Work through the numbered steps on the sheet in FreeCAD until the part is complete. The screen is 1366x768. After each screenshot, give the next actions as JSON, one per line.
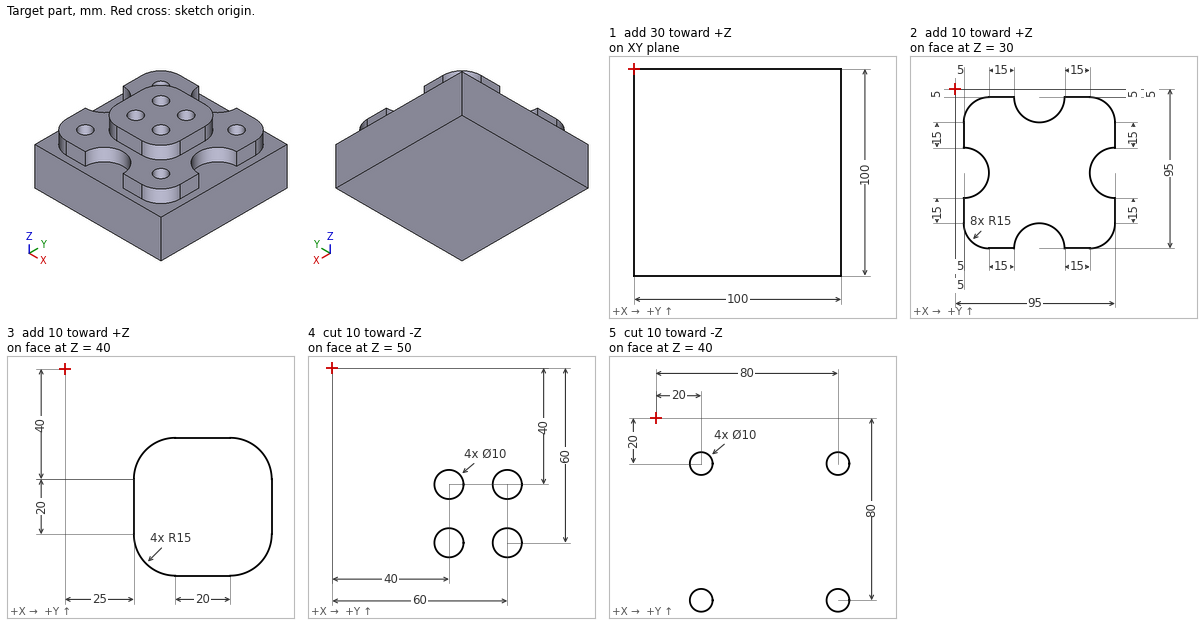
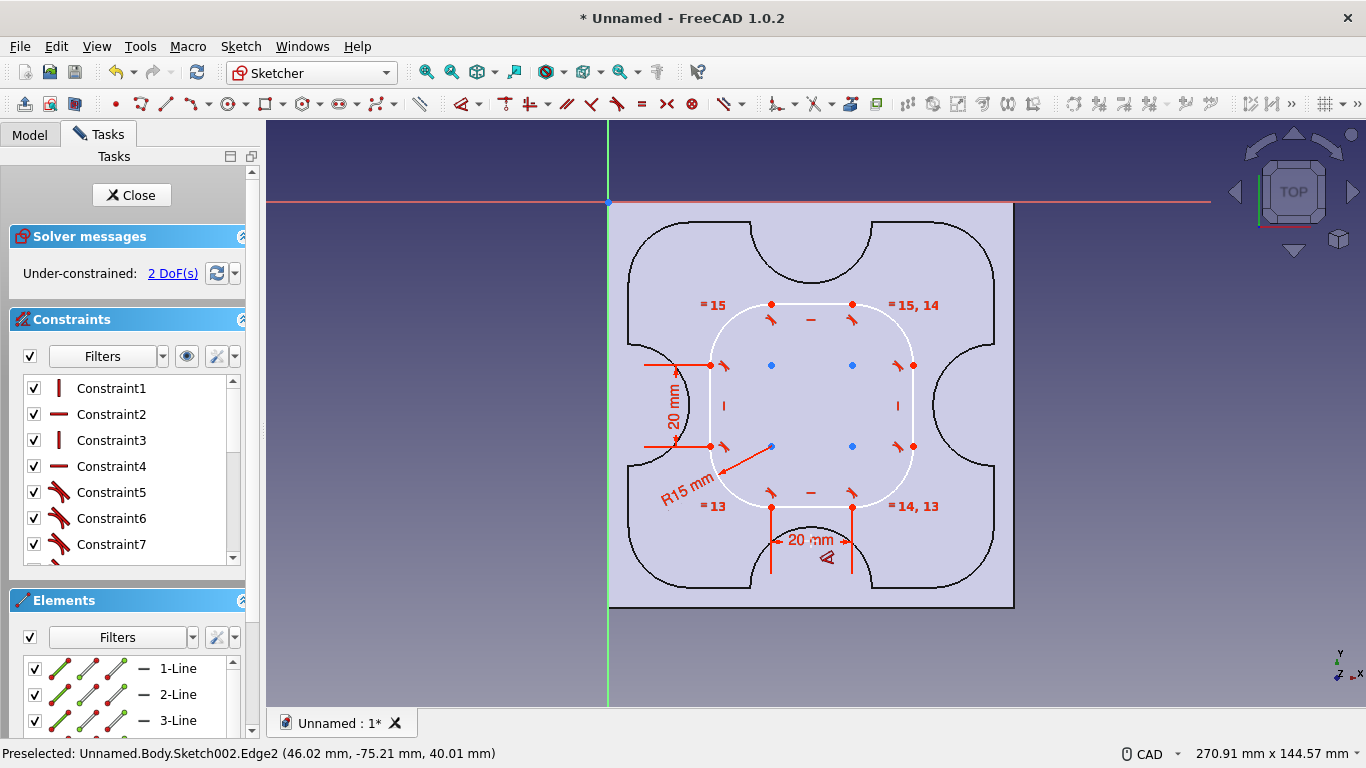
{"action": "left_click", "coordinate": [710, 365]}
{"action": "left_click", "coordinate": [659, 168]}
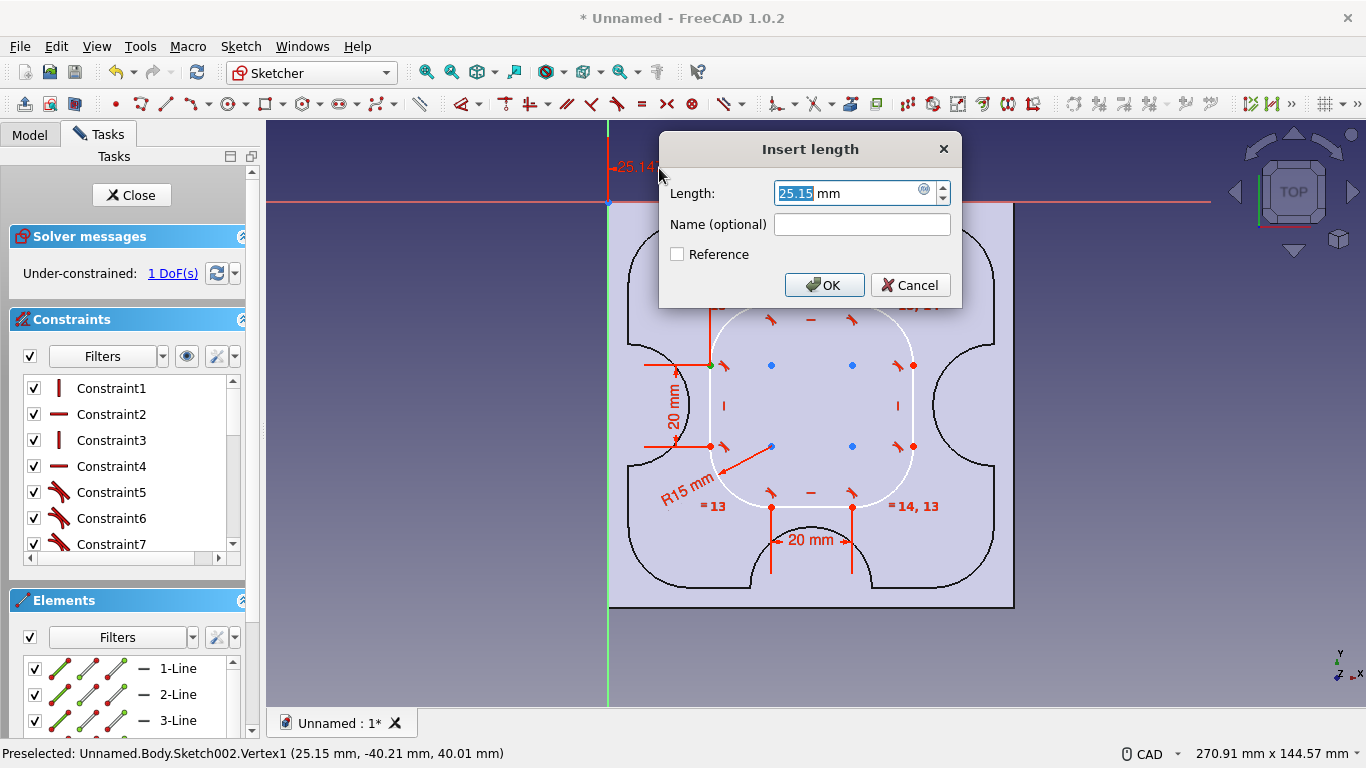
{"action": "type", "text": "25"}
{"action": "key", "text": "Return"}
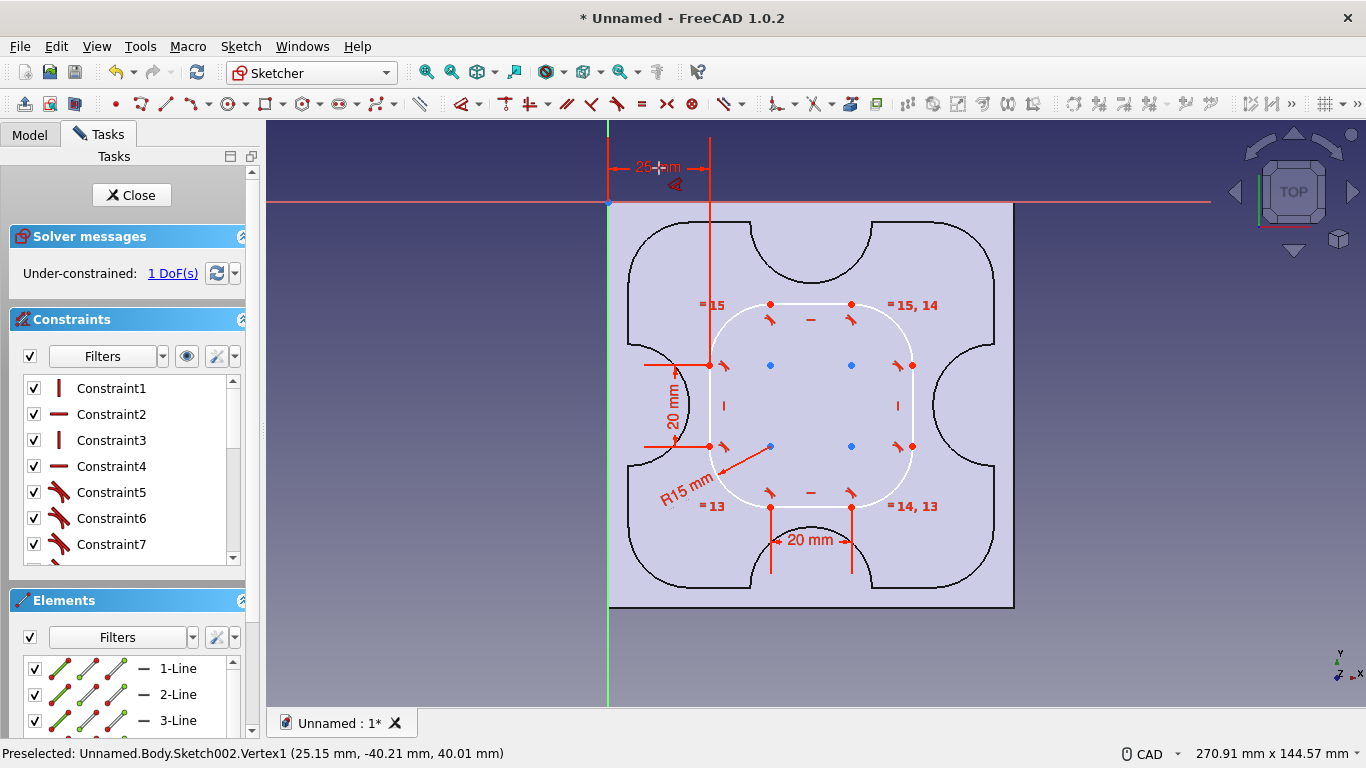
{"action": "left_click", "coordinate": [710, 365]}
{"action": "left_click", "coordinate": [574, 284]}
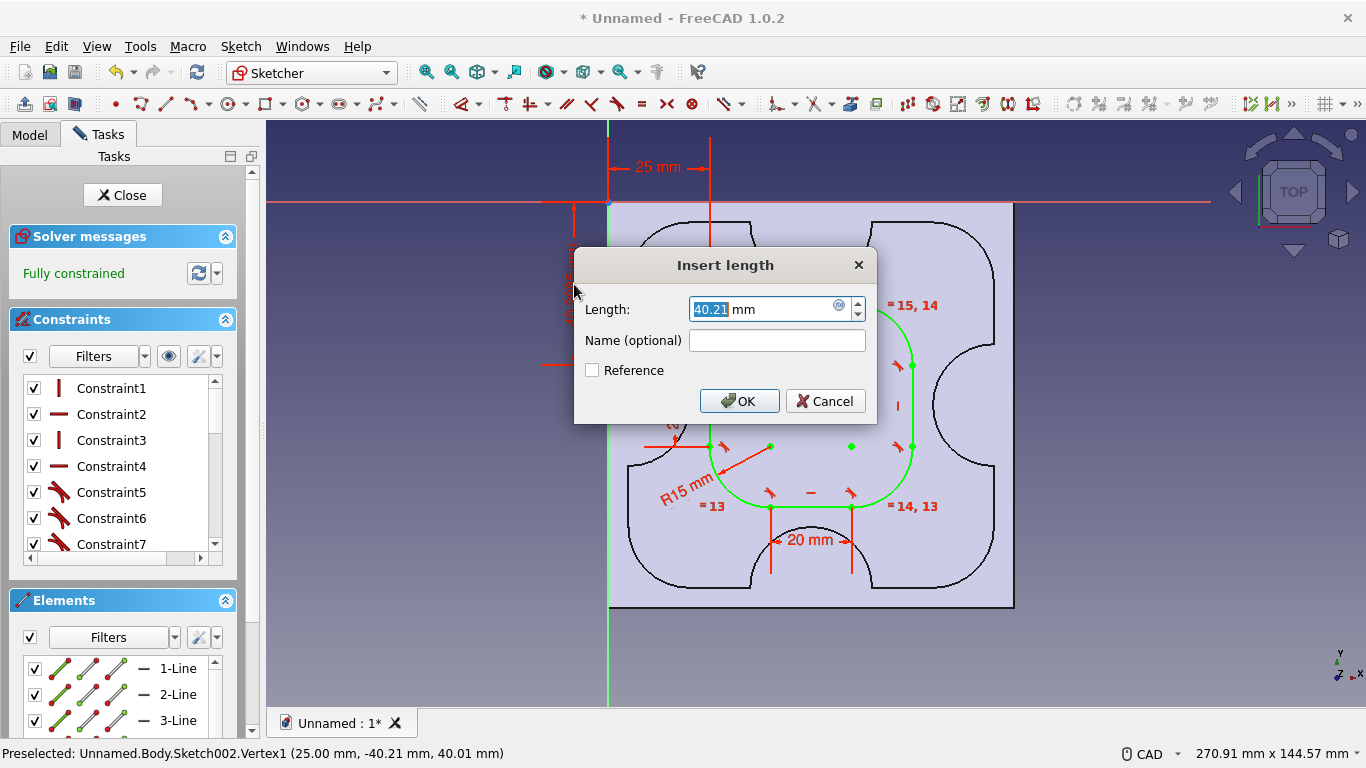
{"action": "type", "text": "40"}
{"action": "key", "text": "Return"}
{"action": "key", "text": "Escape"}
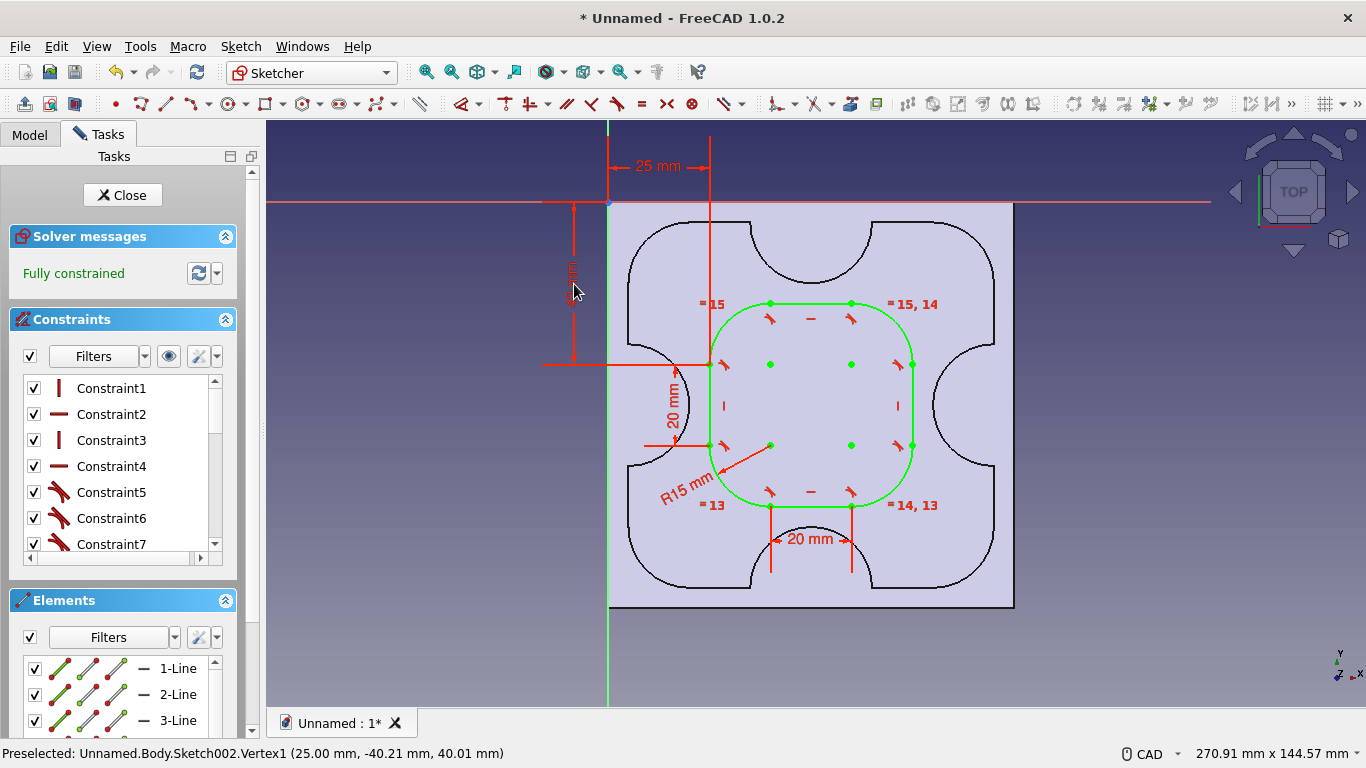
{"action": "left_click", "coordinate": [123, 195]}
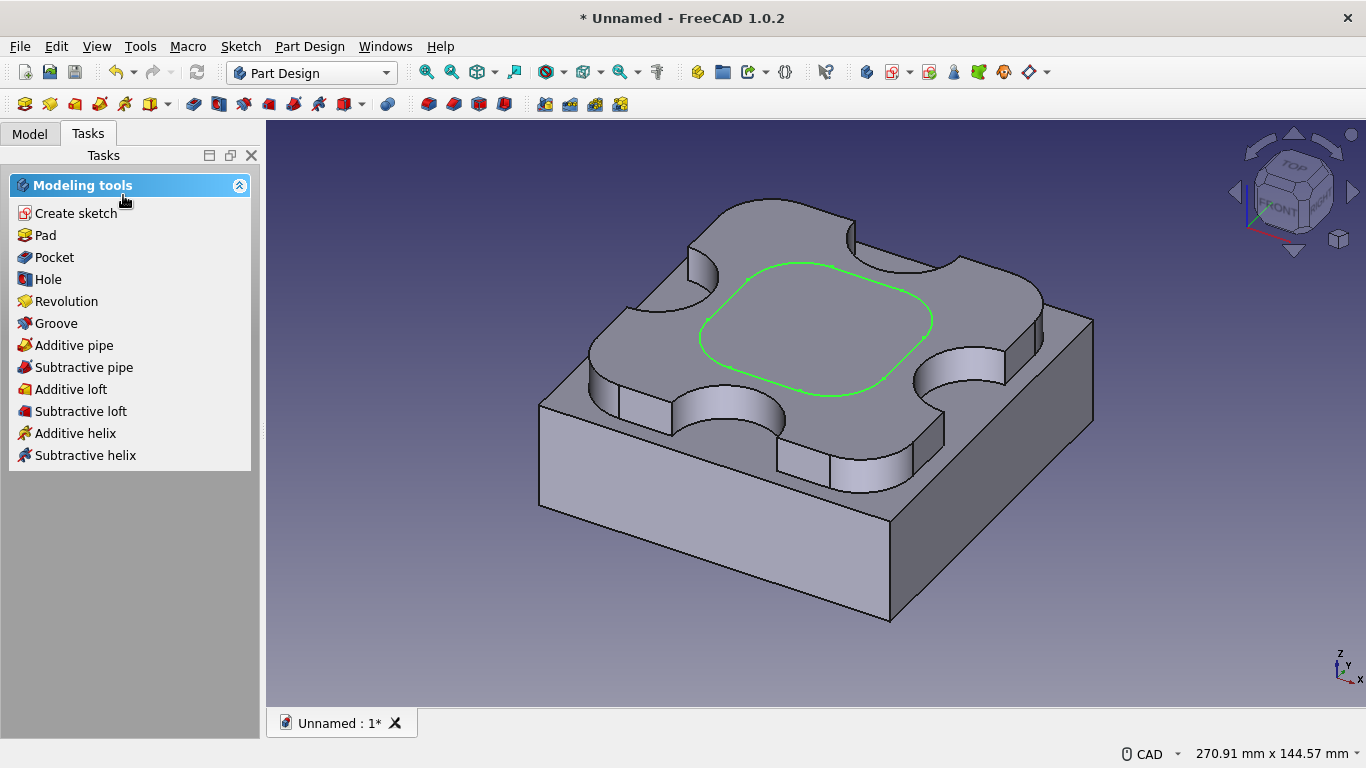
{"action": "left_click", "coordinate": [25, 104]}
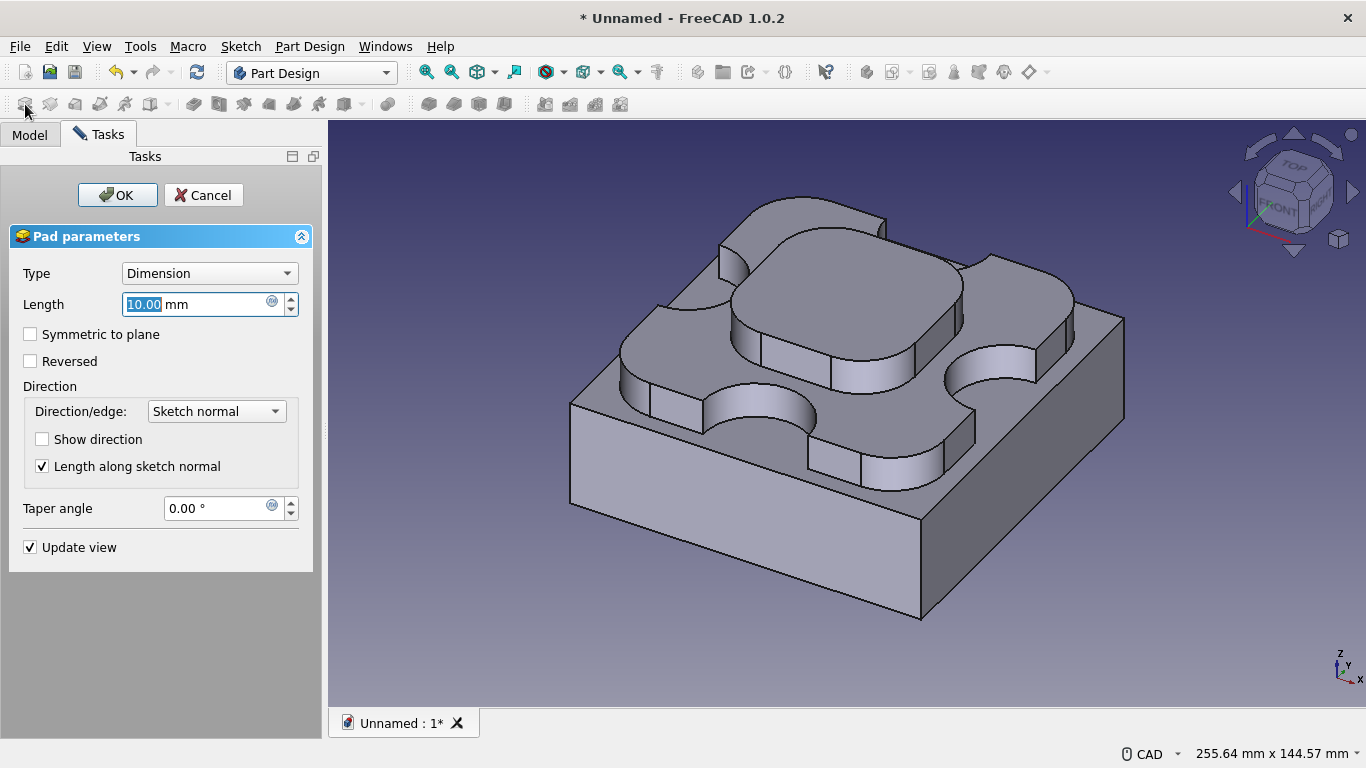
{"action": "type", "text": "10"}
{"action": "key", "text": "Tab"}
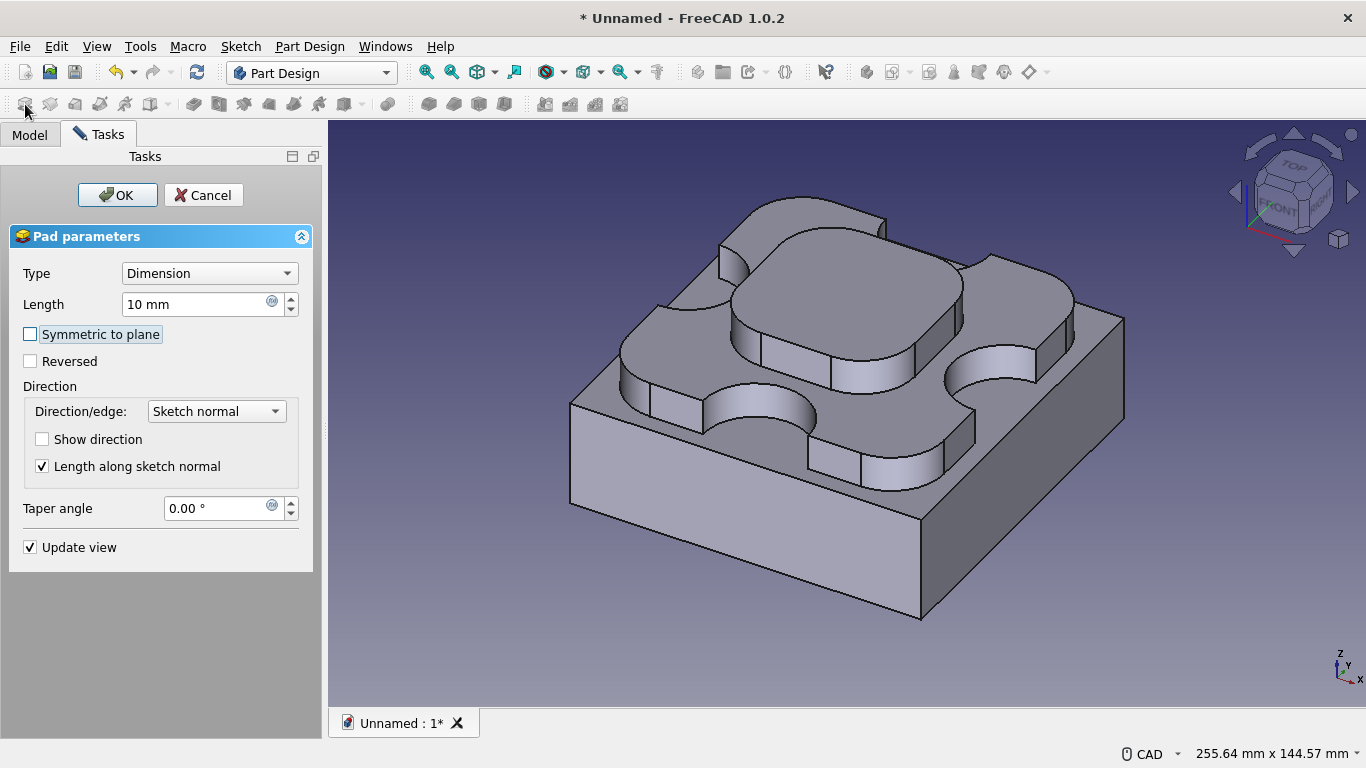
{"action": "left_click", "coordinate": [118, 195]}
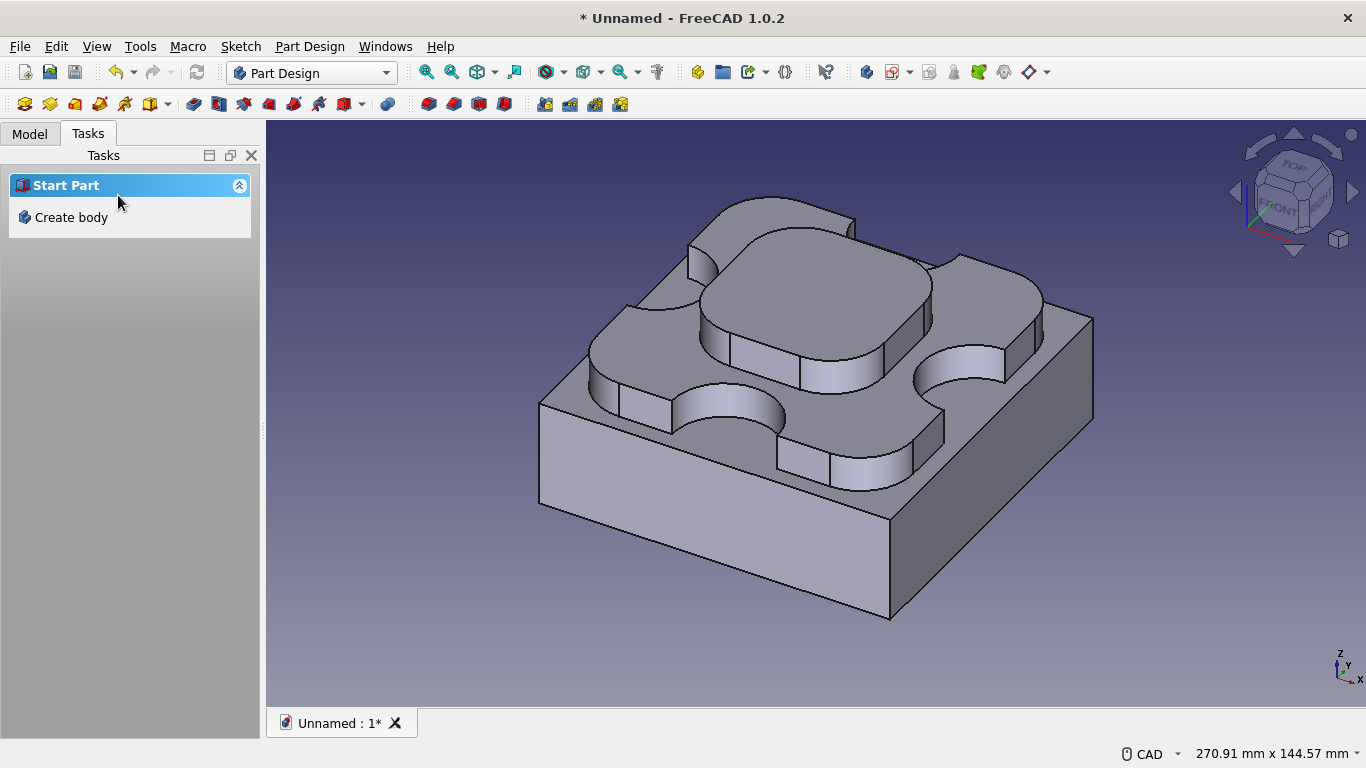
{"action": "left_click", "coordinate": [816, 293]}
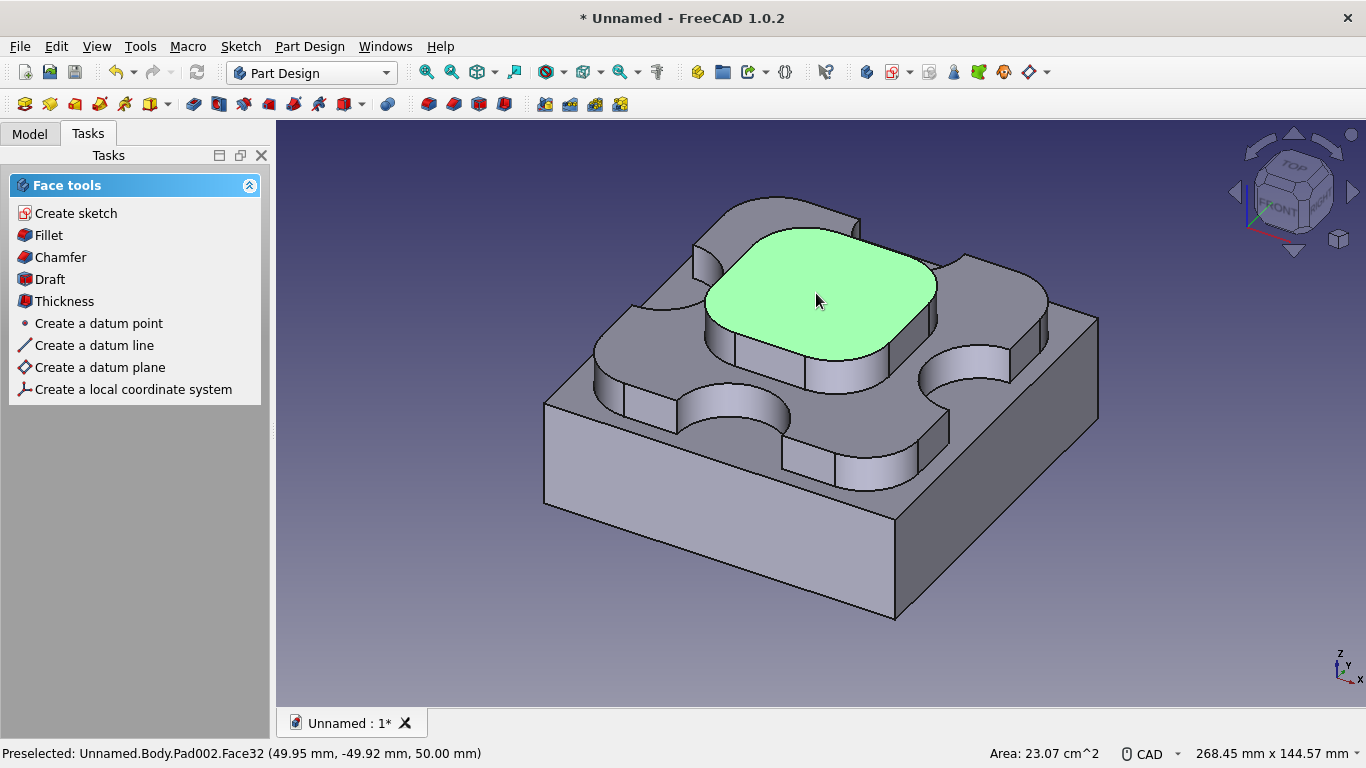
{"action": "left_click", "coordinate": [892, 72]}